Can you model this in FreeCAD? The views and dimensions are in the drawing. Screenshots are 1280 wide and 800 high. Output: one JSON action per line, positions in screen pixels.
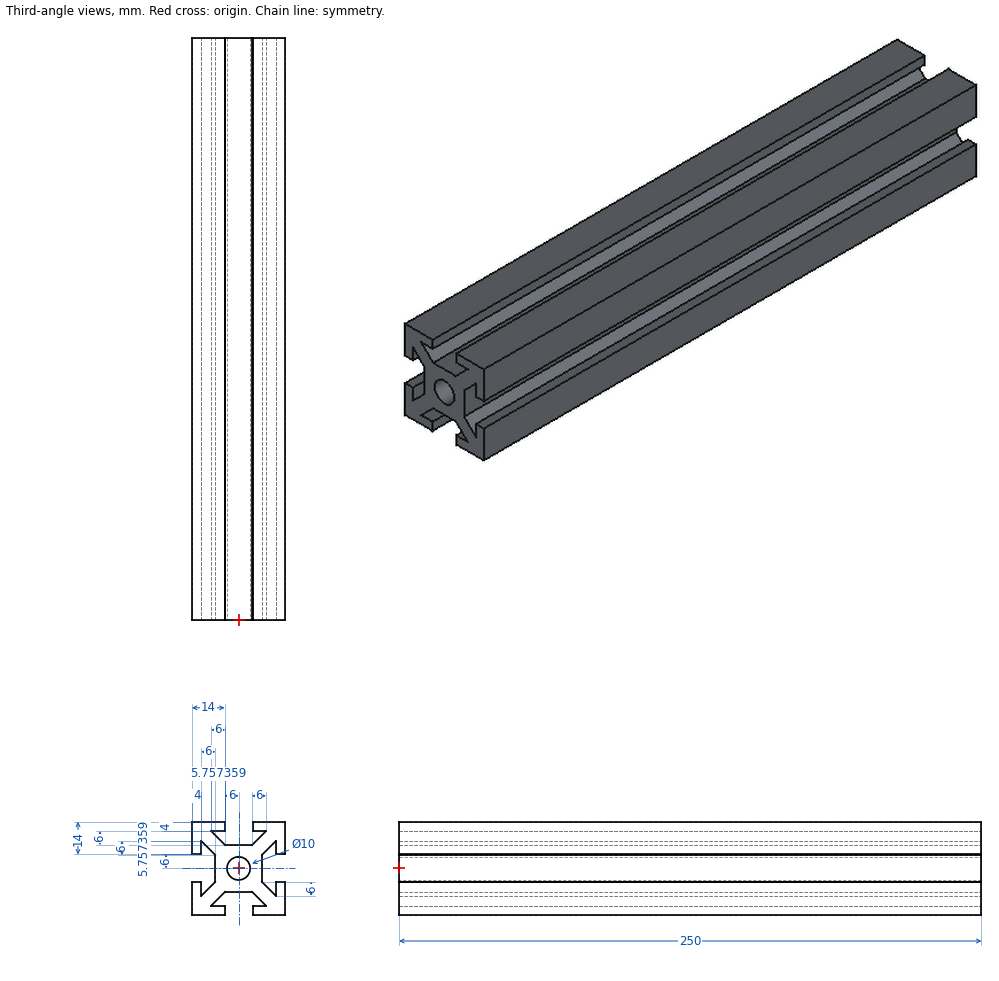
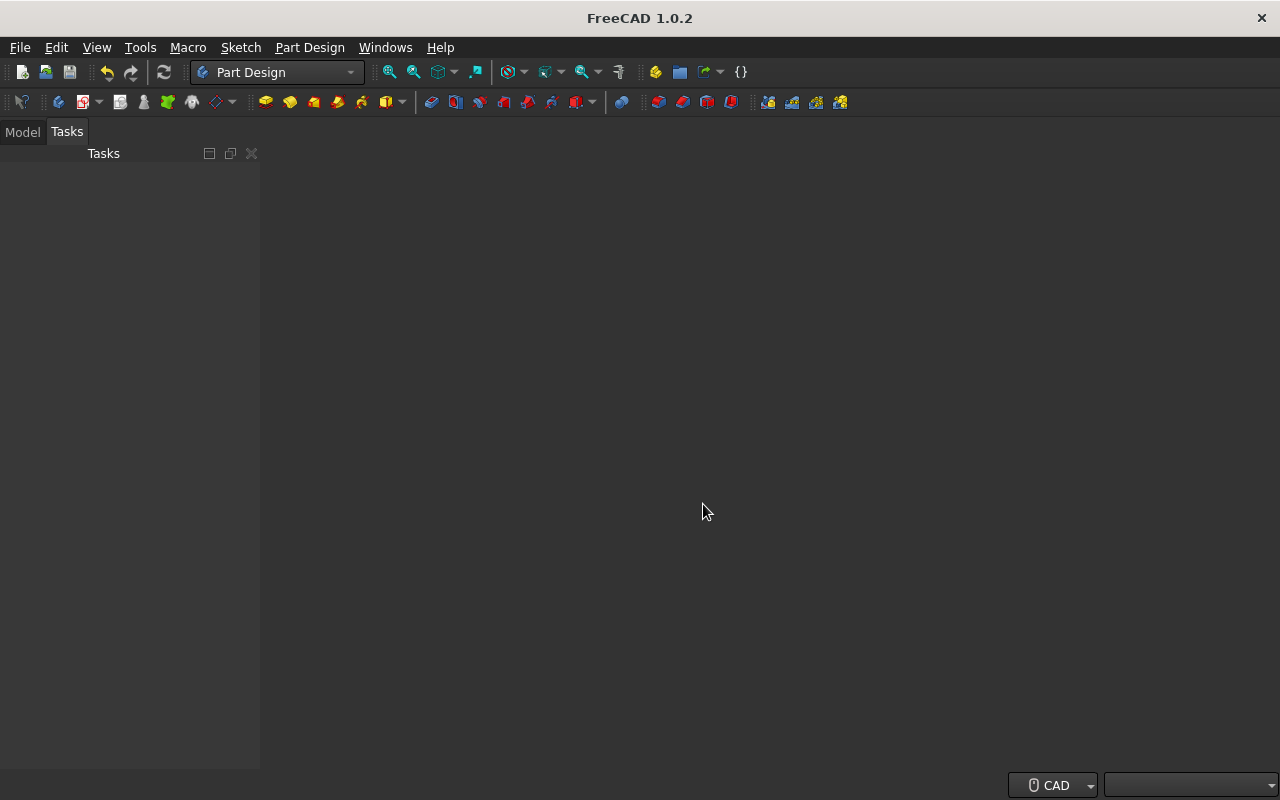
{"action": "left_click", "coordinate": [22, 72]}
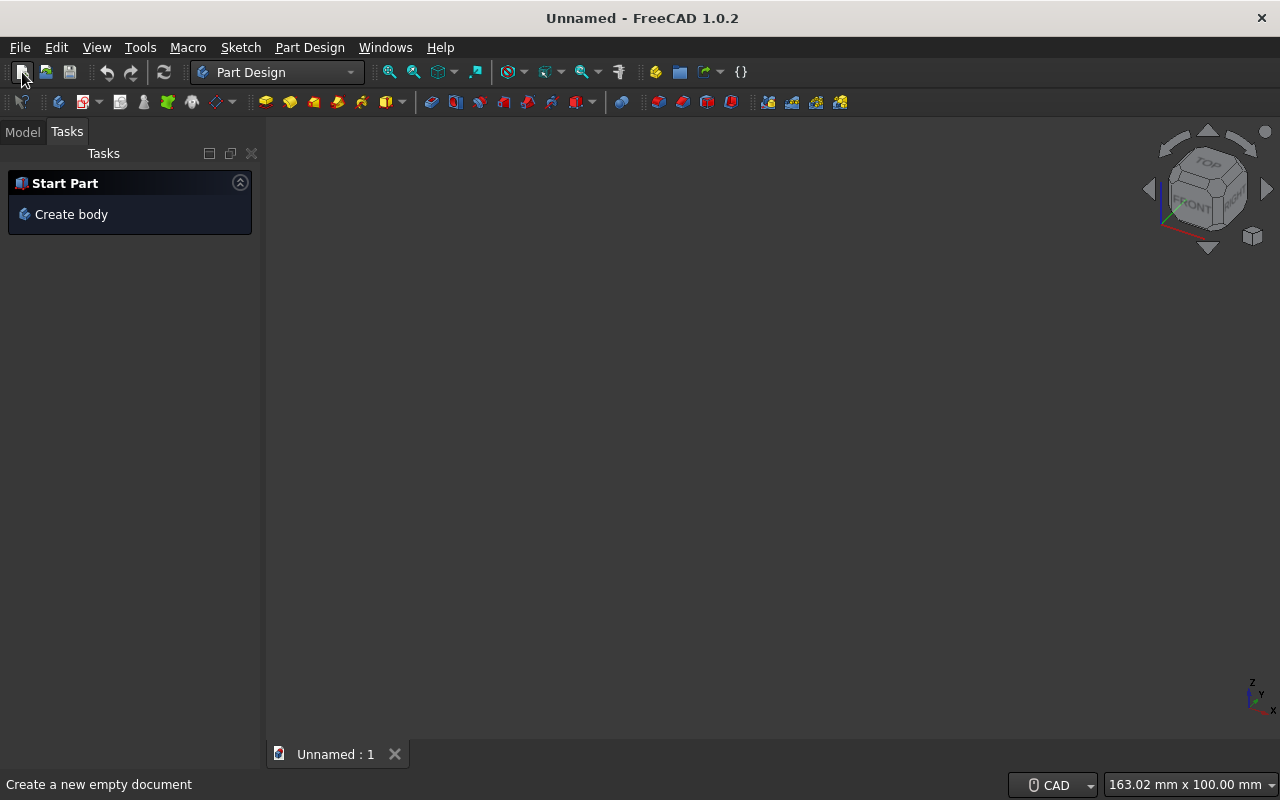
{"action": "left_click", "coordinate": [84, 102]}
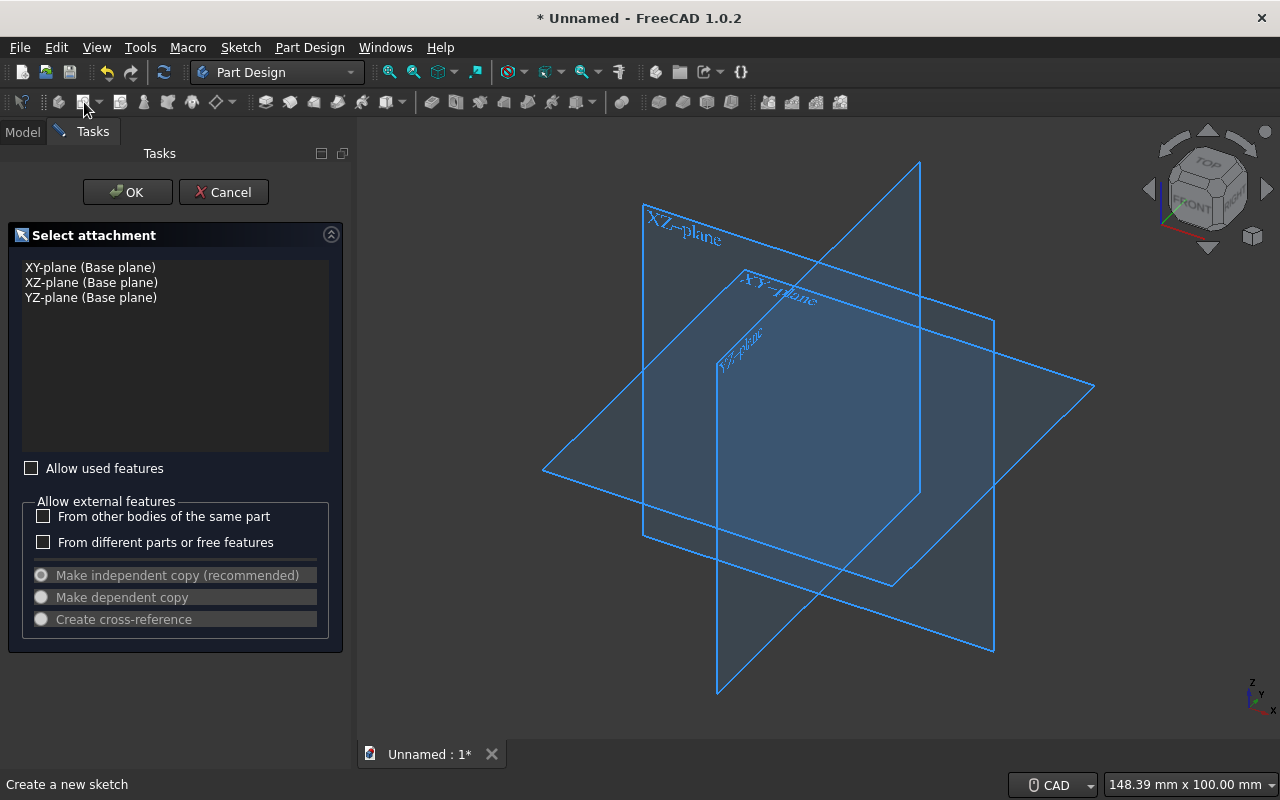
{"action": "left_click", "coordinate": [82, 282]}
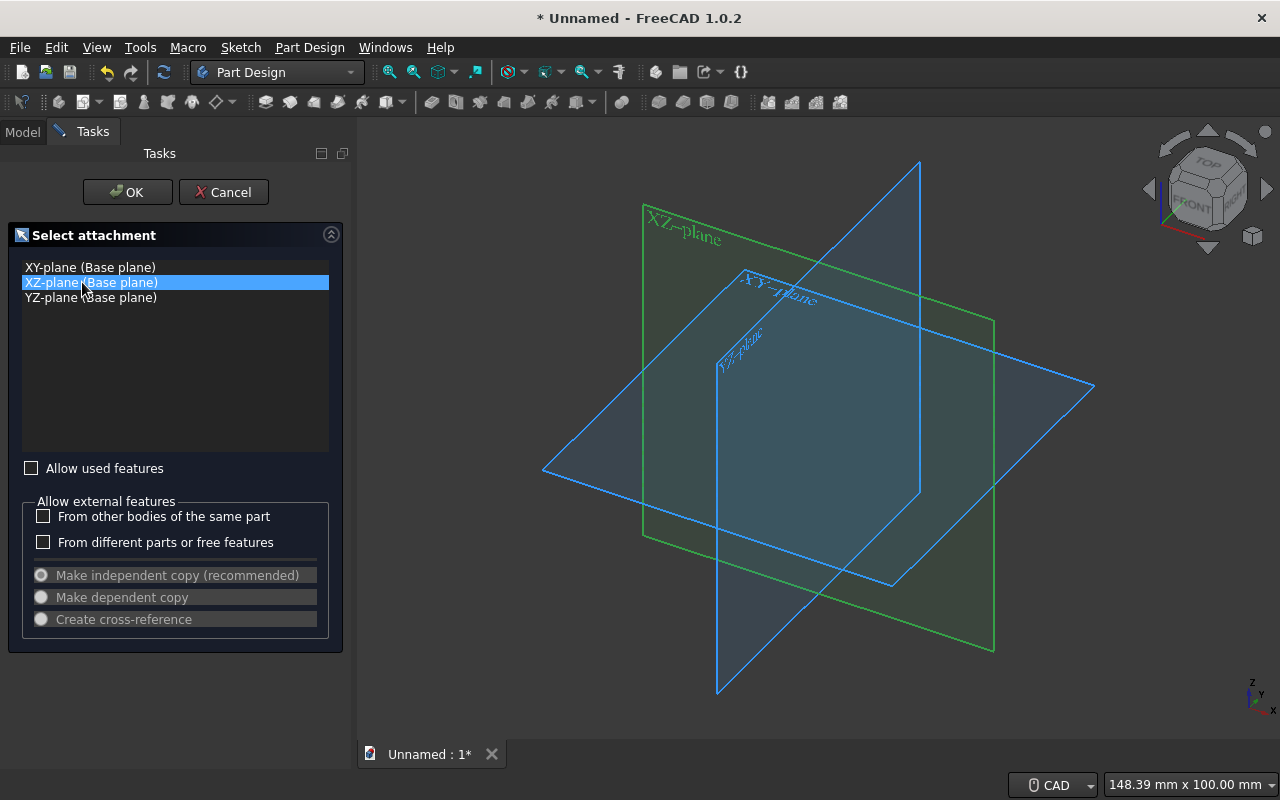
{"action": "left_click", "coordinate": [128, 192]}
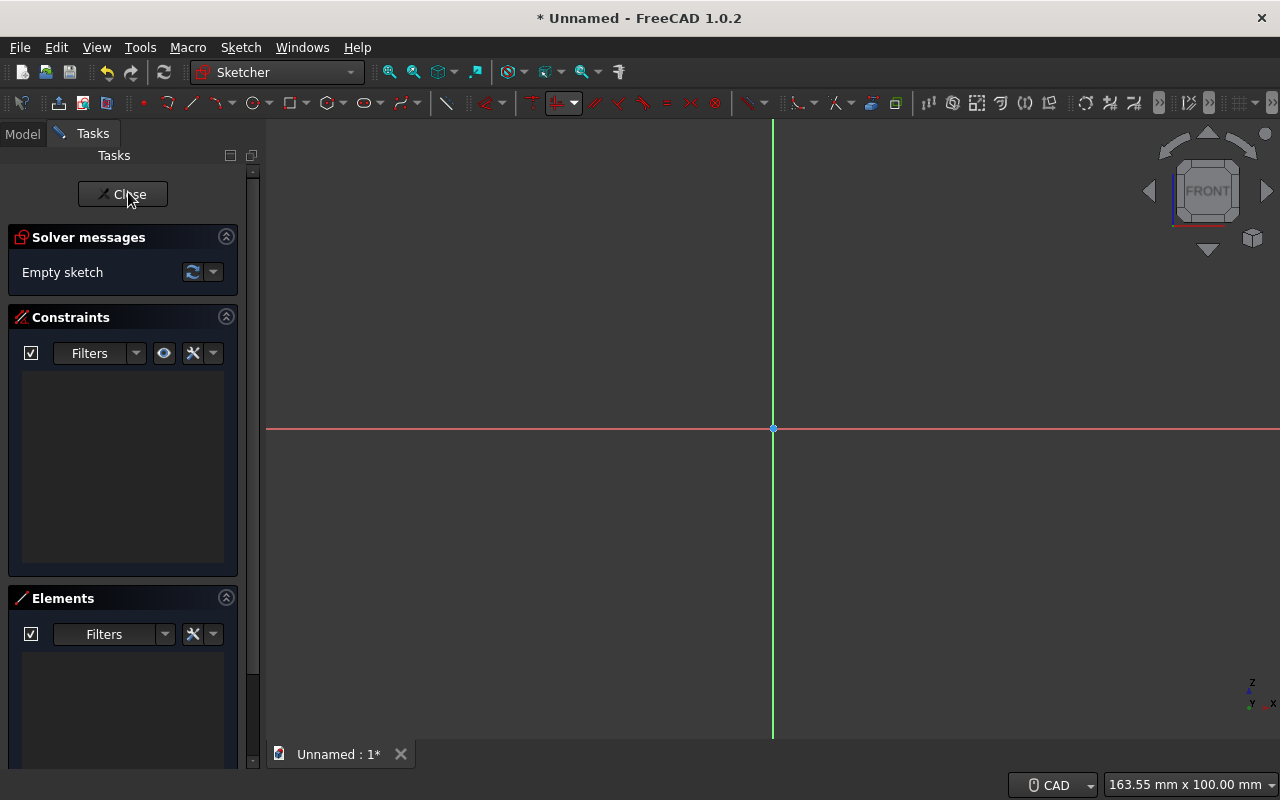
{"action": "scroll", "coordinate": [912, 429], "scroll_direction": "up", "scroll_amount": 2}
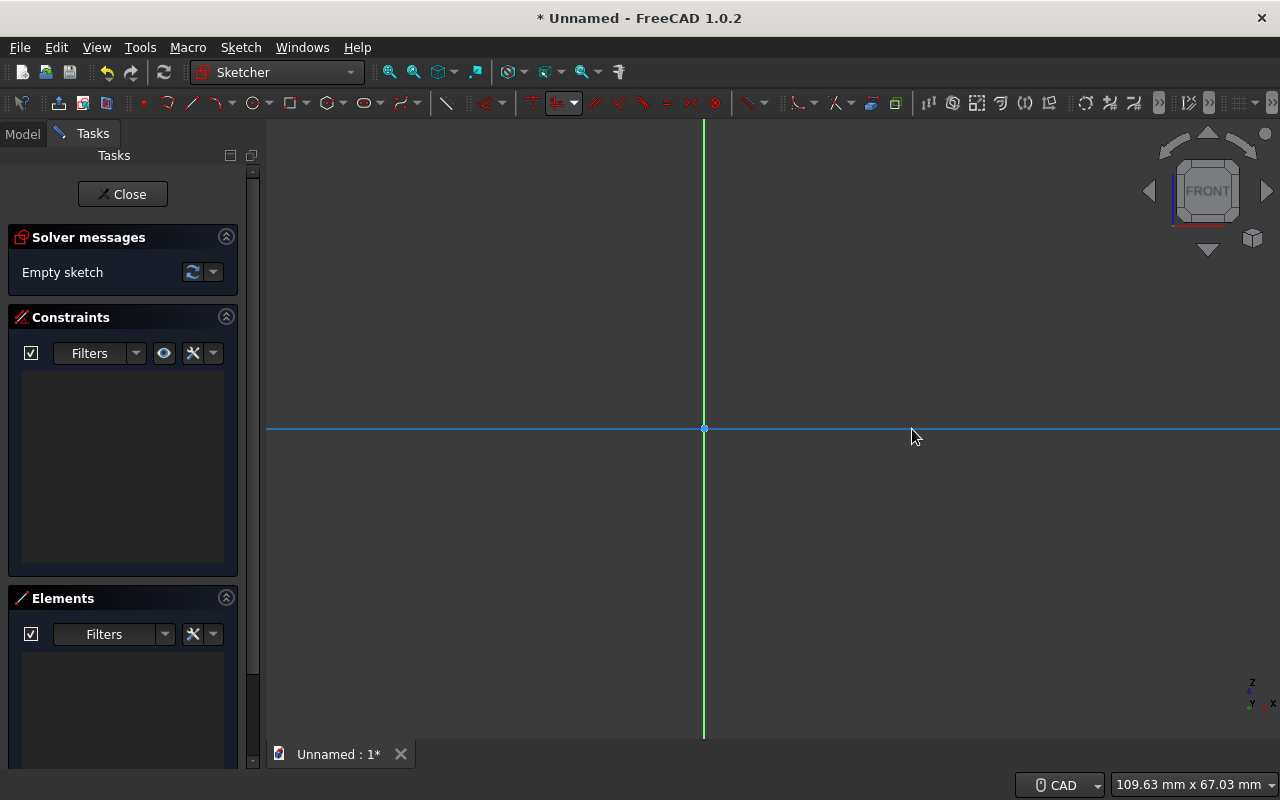
{"action": "left_click", "coordinate": [168, 104]}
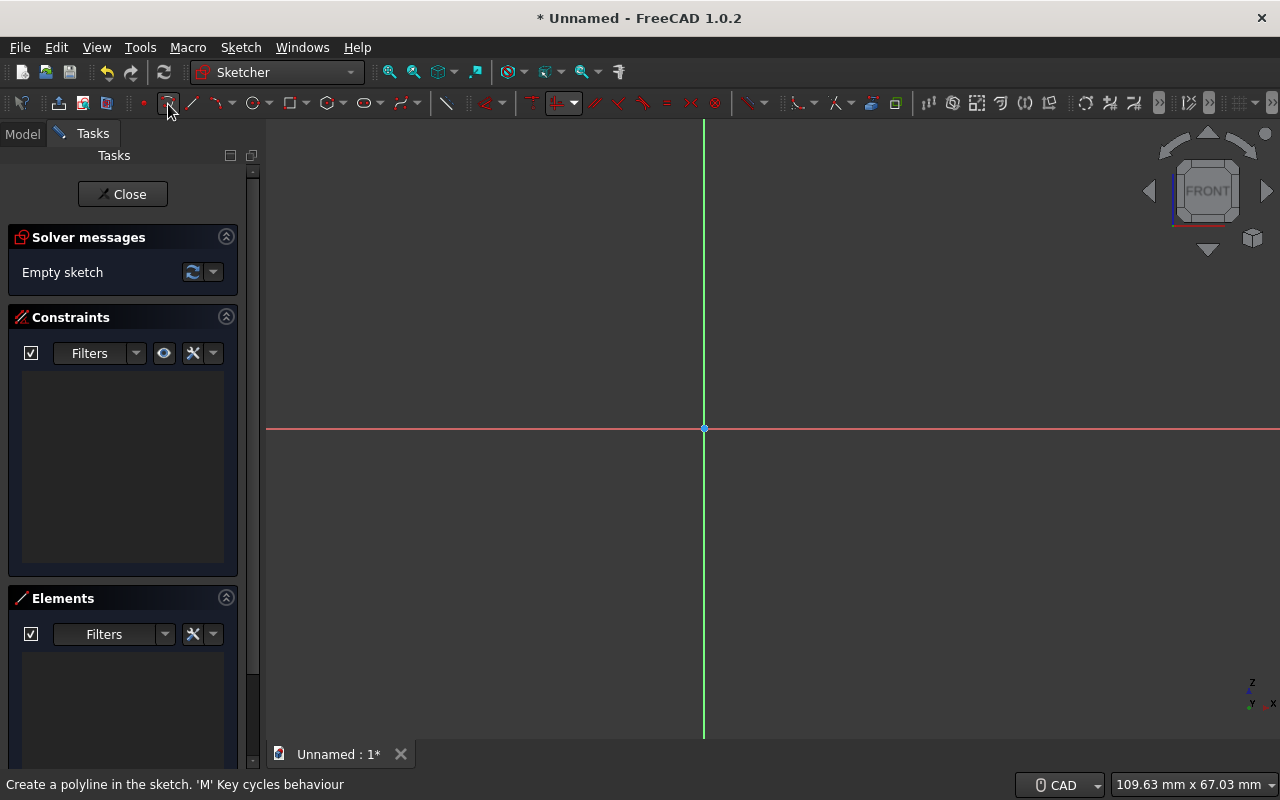
{"action": "left_click", "coordinate": [612, 482]}
{"action": "left_click", "coordinate": [612, 376]}
{"action": "left_click", "coordinate": [556, 320]}
{"action": "left_click", "coordinate": [556, 373]}
{"action": "left_click", "coordinate": [519, 373]}
{"action": "left_click", "coordinate": [519, 244]}
{"action": "left_click", "coordinate": [649, 244]}
{"action": "left_click", "coordinate": [649, 281]}
{"action": "left_click", "coordinate": [596, 281]}
{"action": "left_click", "coordinate": [651, 336]}
{"action": "left_click", "coordinate": [758, 336]}
{"action": "left_click", "coordinate": [813, 281]}
{"action": "left_click", "coordinate": [760, 281]}
{"action": "left_click", "coordinate": [760, 244]}
{"action": "left_click", "coordinate": [889, 244]}
{"action": "left_click", "coordinate": [889, 373]}
{"action": "left_click", "coordinate": [852, 373]}
{"action": "left_click", "coordinate": [852, 320]}
{"action": "left_click", "coordinate": [797, 376]}
{"action": "left_click", "coordinate": [797, 482]}
{"action": "left_click", "coordinate": [852, 538]}
{"action": "left_click", "coordinate": [852, 484]}
{"action": "left_click", "coordinate": [889, 484]}
{"action": "left_click", "coordinate": [889, 614]}
{"action": "left_click", "coordinate": [760, 614]}
{"action": "left_click", "coordinate": [760, 577]}
{"action": "left_click", "coordinate": [813, 577]}
{"action": "left_click", "coordinate": [758, 521]}
{"action": "left_click", "coordinate": [651, 521]}
{"action": "left_click", "coordinate": [596, 577]}
{"action": "left_click", "coordinate": [649, 577]}
{"action": "left_click", "coordinate": [649, 614]}
{"action": "left_click", "coordinate": [519, 614]}
{"action": "left_click", "coordinate": [519, 484]}
{"action": "left_click", "coordinate": [556, 484]}
{"action": "left_click", "coordinate": [556, 538]}
{"action": "left_click", "coordinate": [612, 483]}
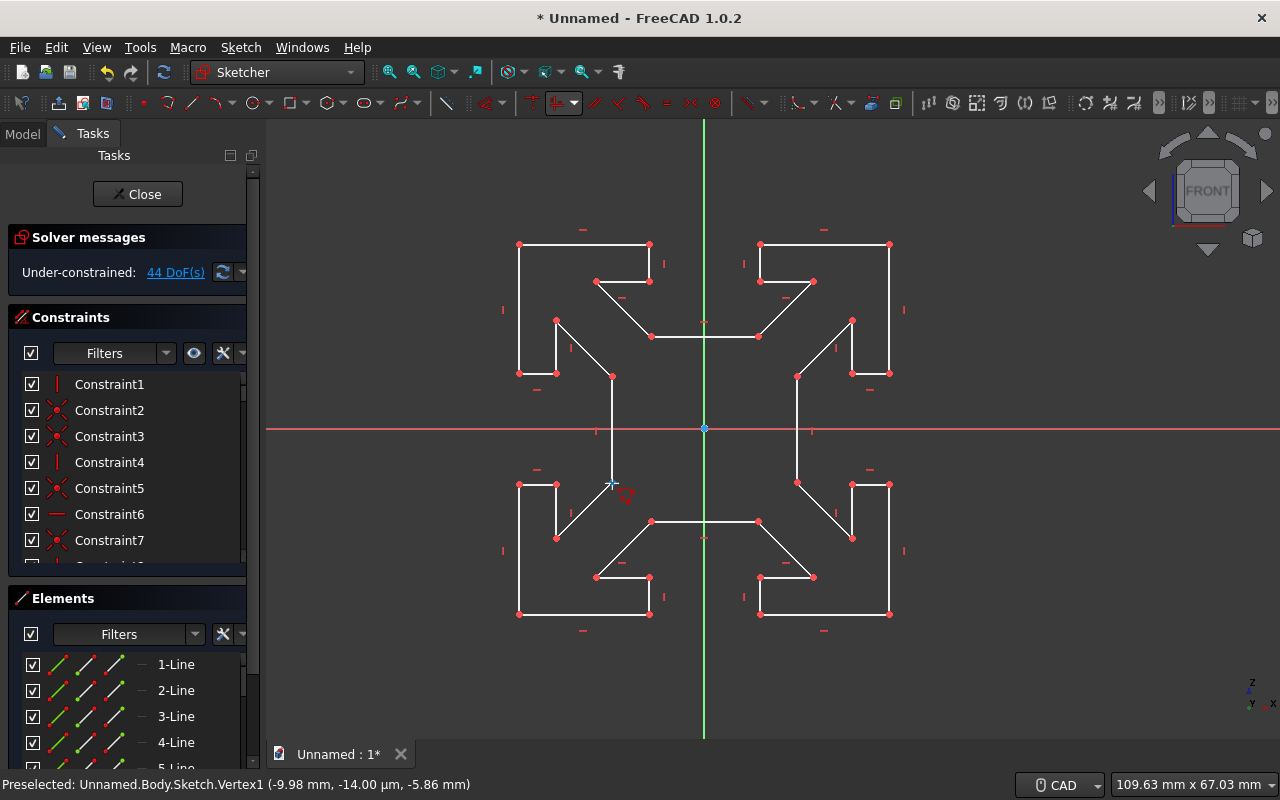
{"action": "left_click", "coordinate": [254, 104]}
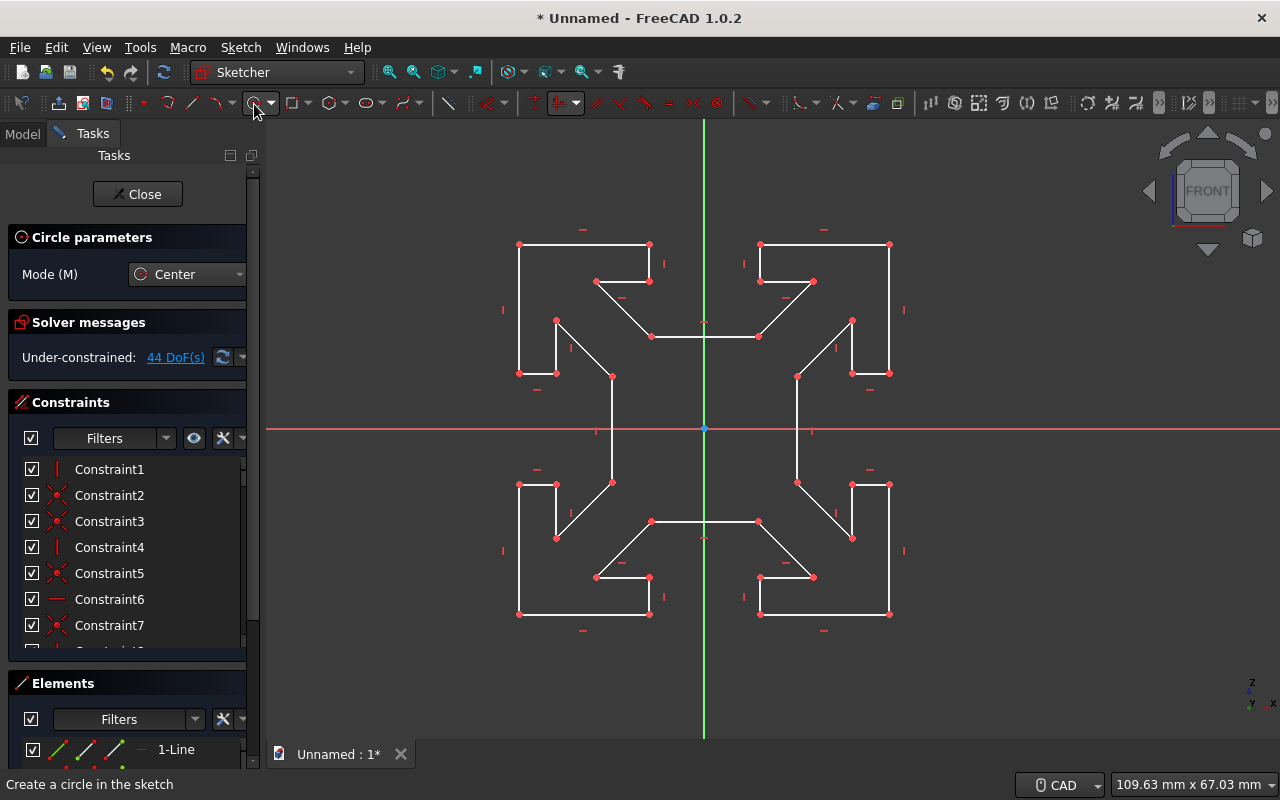
{"action": "left_click", "coordinate": [704, 429]}
{"action": "mouse_move", "coordinate": [737, 396]}